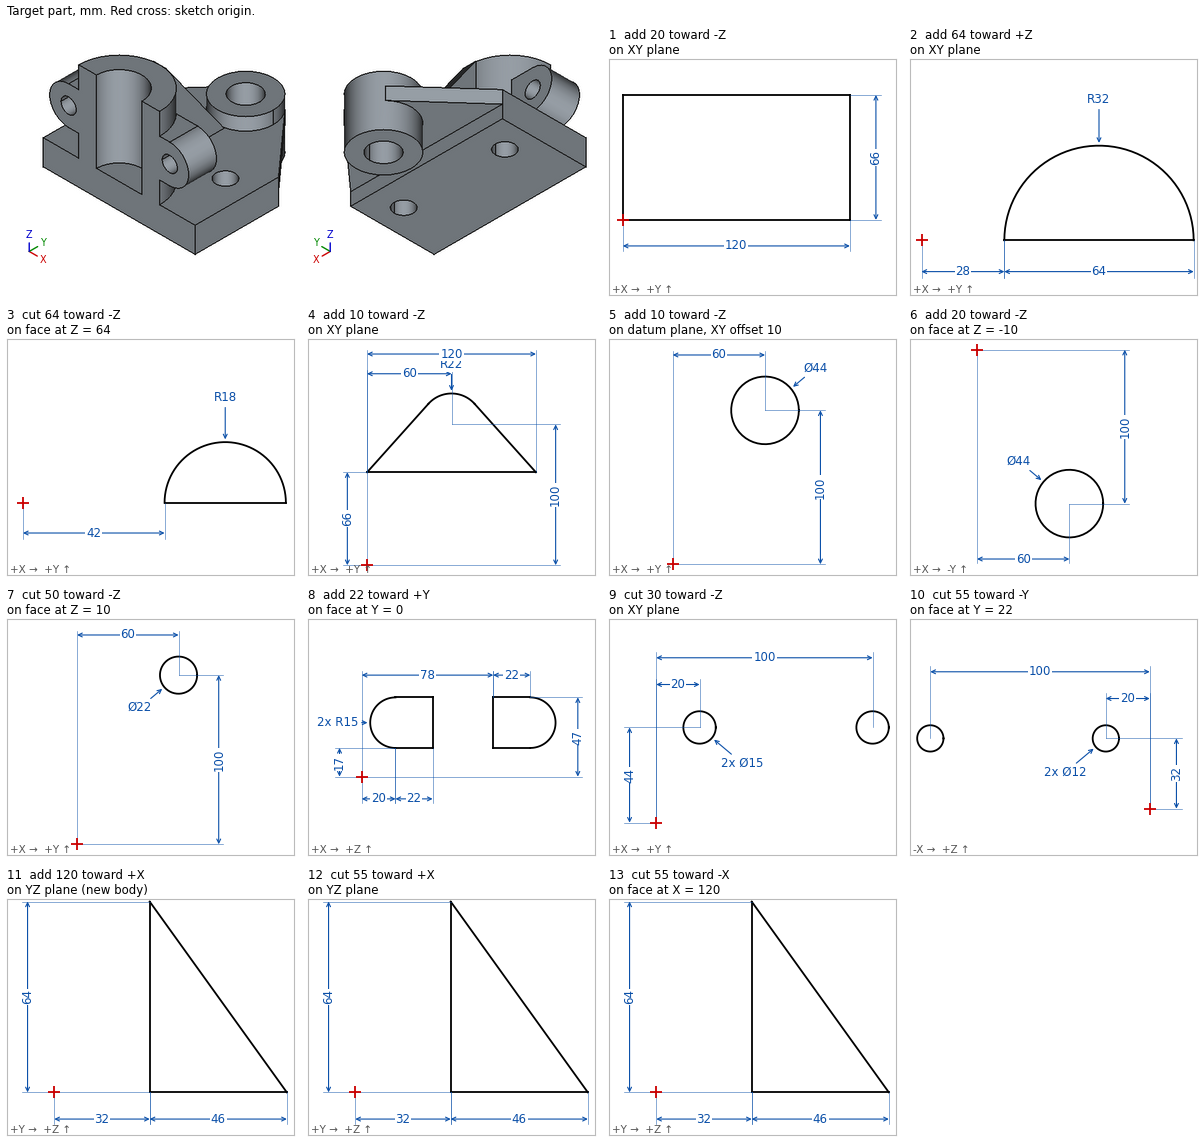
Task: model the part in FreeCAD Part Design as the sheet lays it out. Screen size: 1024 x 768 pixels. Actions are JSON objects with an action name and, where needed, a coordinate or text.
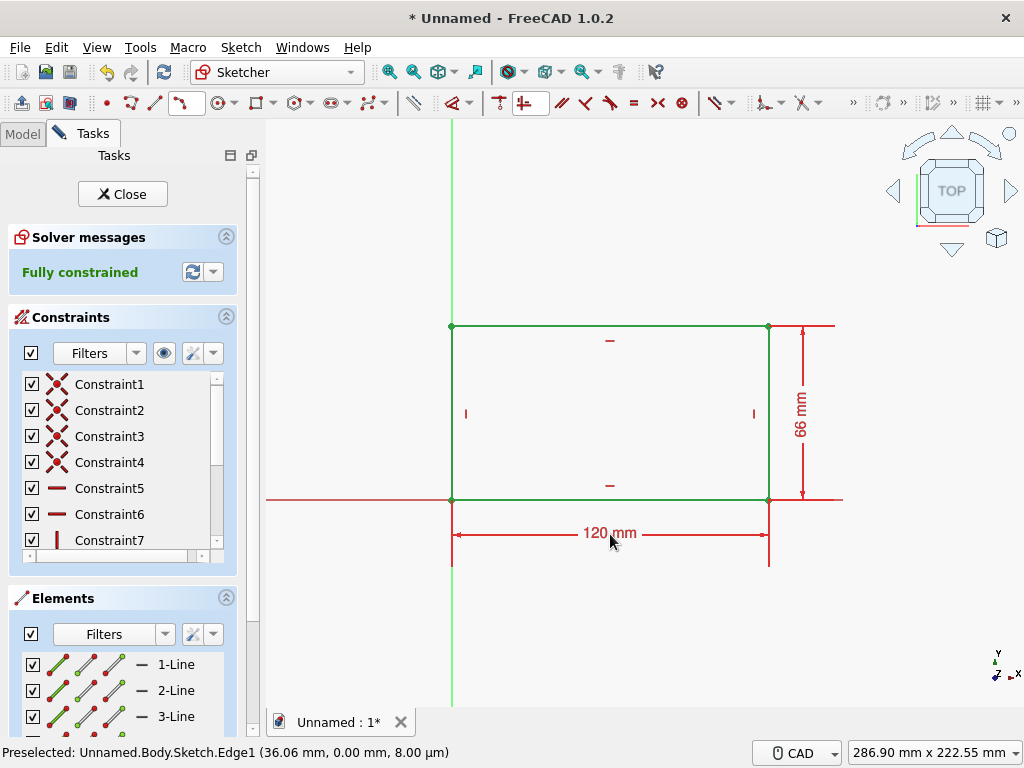
{"action": "left_click", "coordinate": [123, 194]}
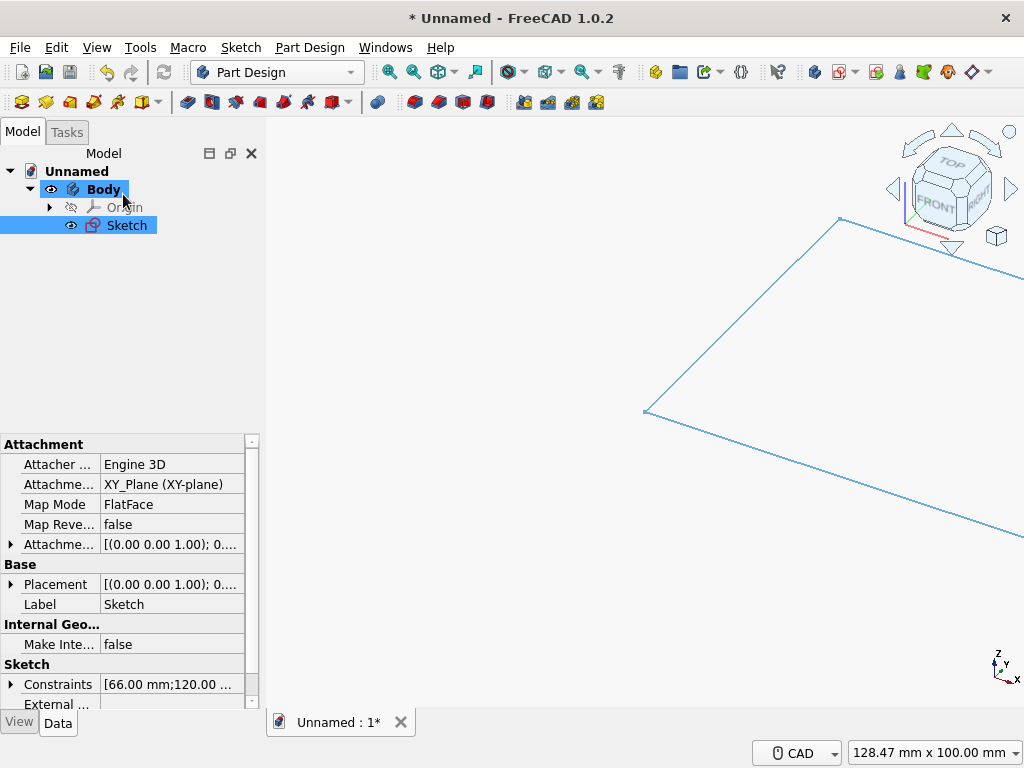
{"action": "left_click", "coordinate": [22, 102]}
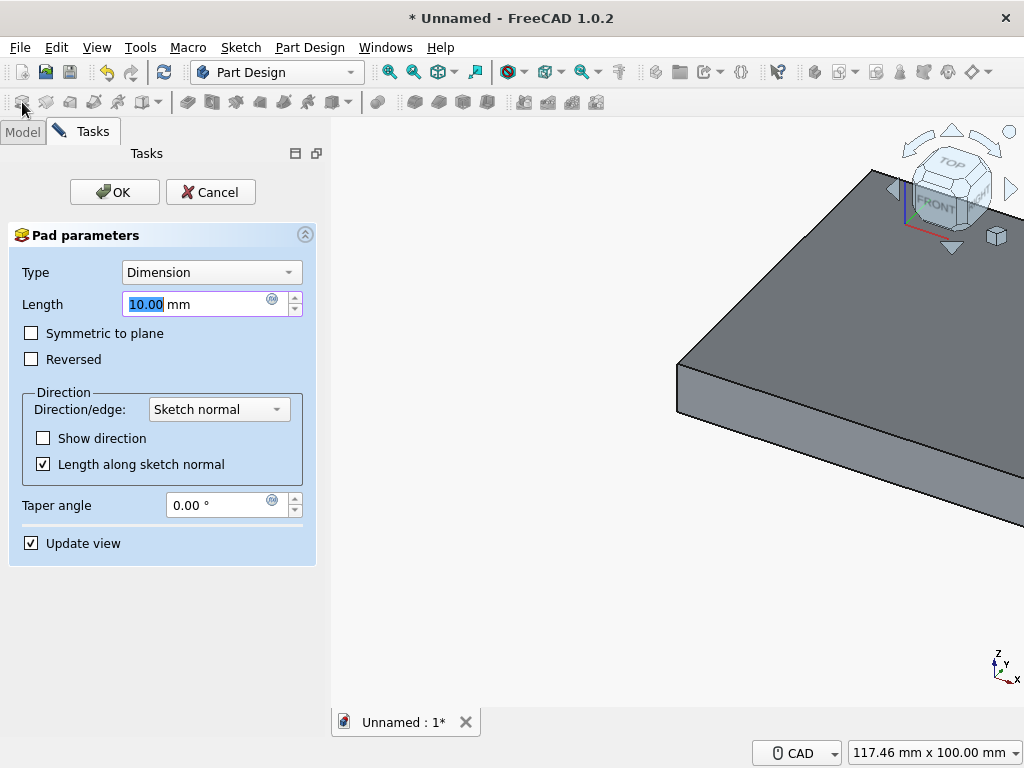
{"action": "type", "text": "20"}
{"action": "key", "text": "Tab"}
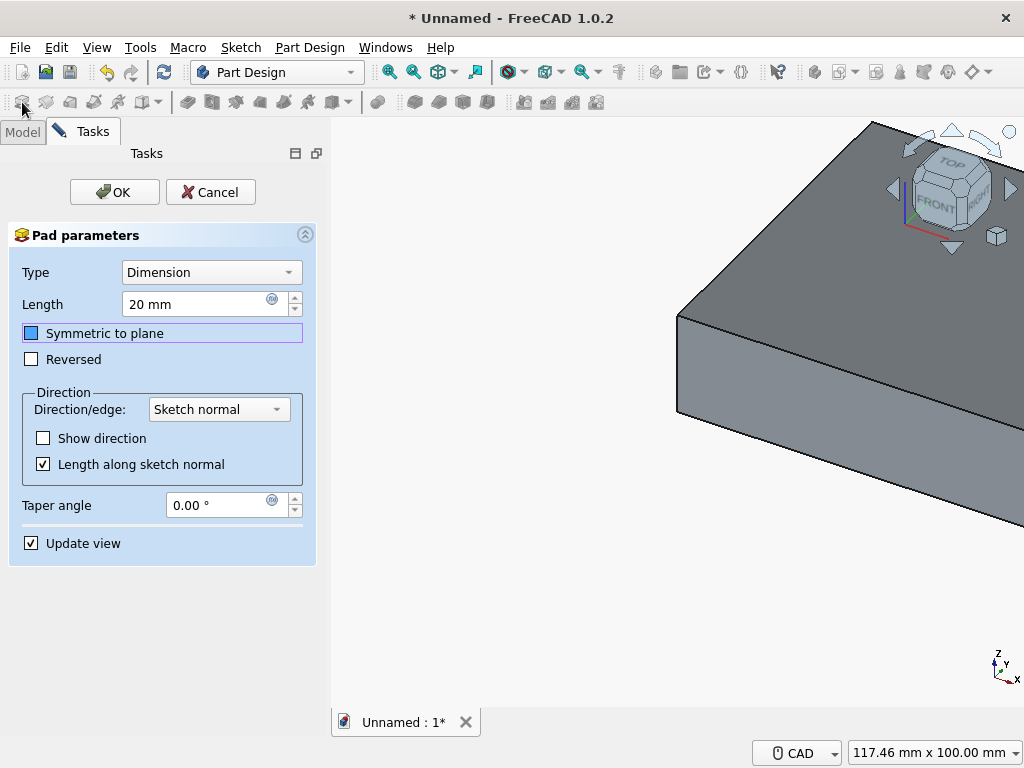
{"action": "left_click", "coordinate": [30, 359]}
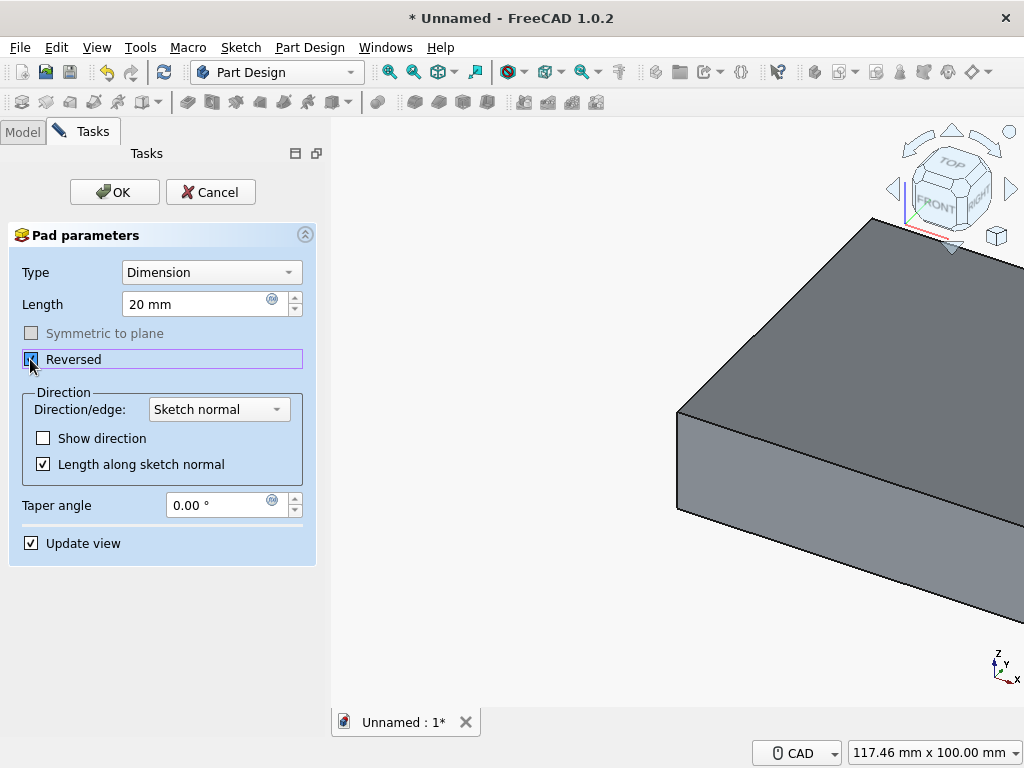
{"action": "left_click", "coordinate": [115, 192]}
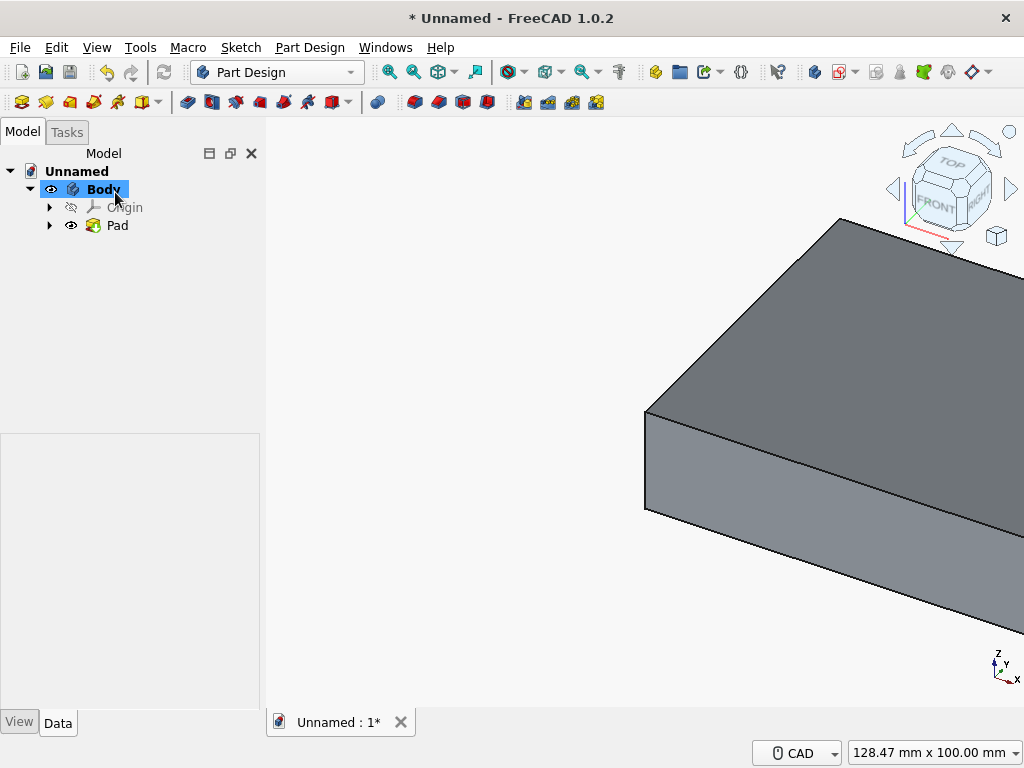
{"action": "left_click", "coordinate": [390, 72]}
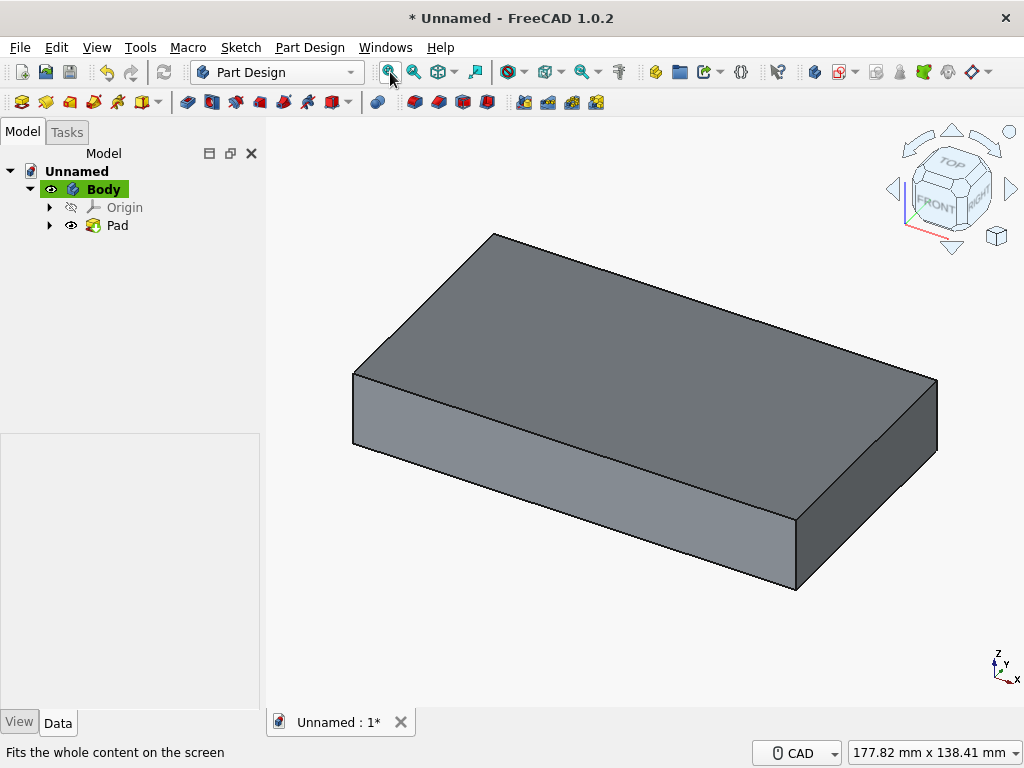
{"action": "left_click", "coordinate": [840, 72]}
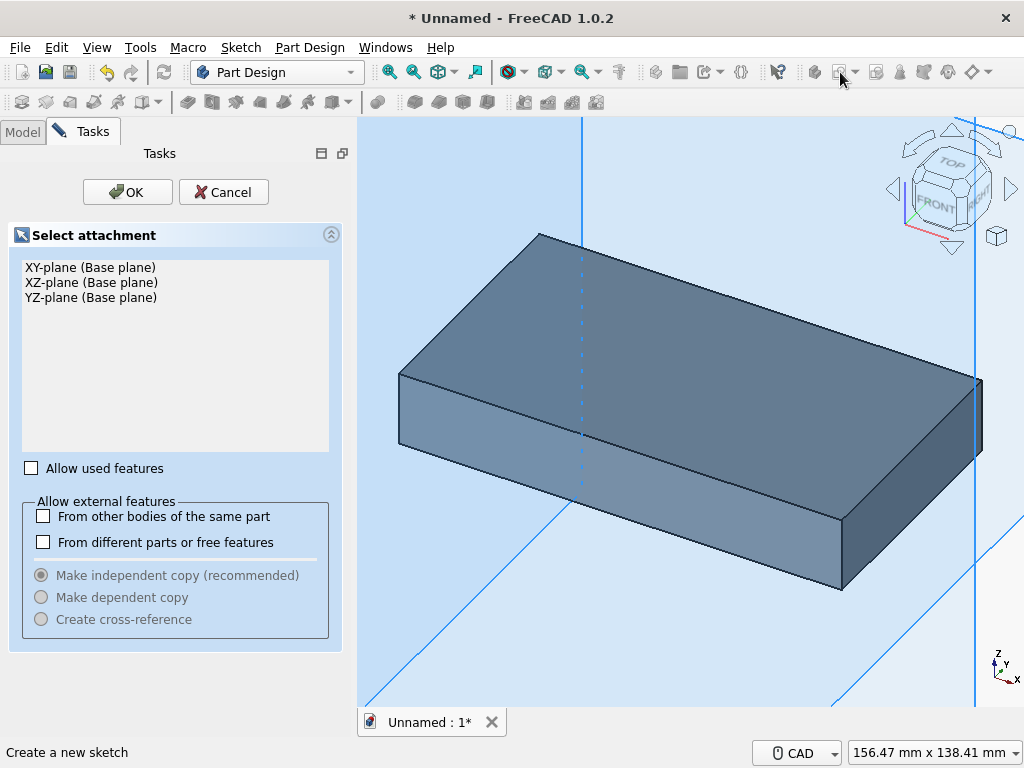
{"action": "left_click", "coordinate": [82, 268]}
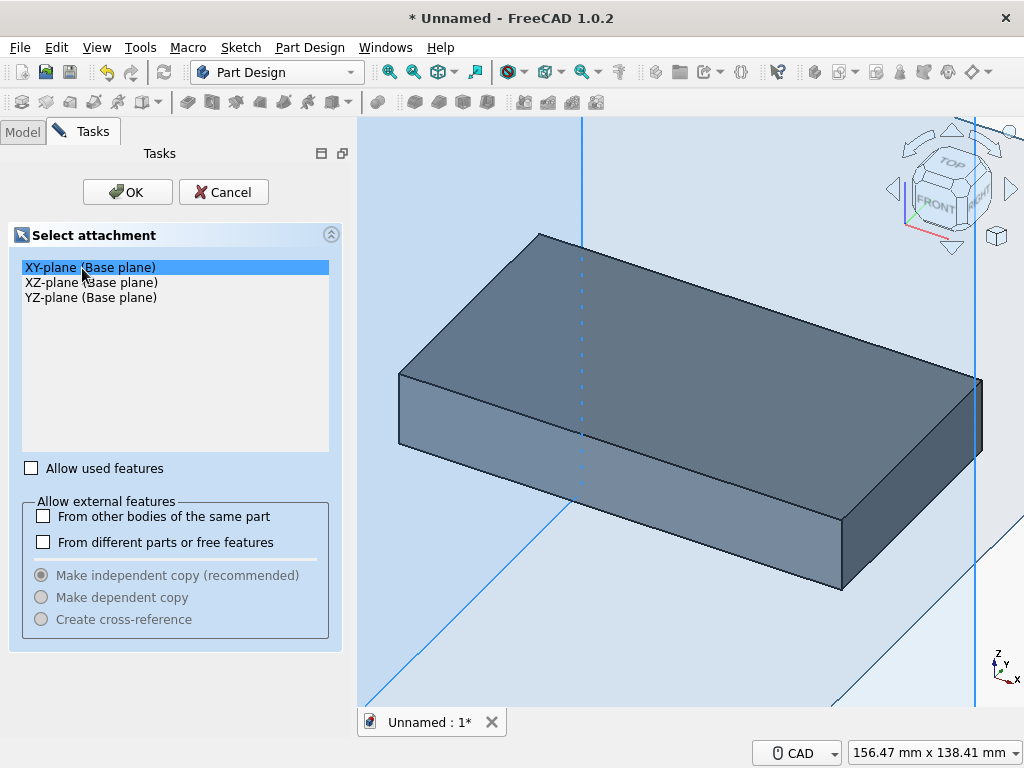
{"action": "left_click", "coordinate": [128, 192]}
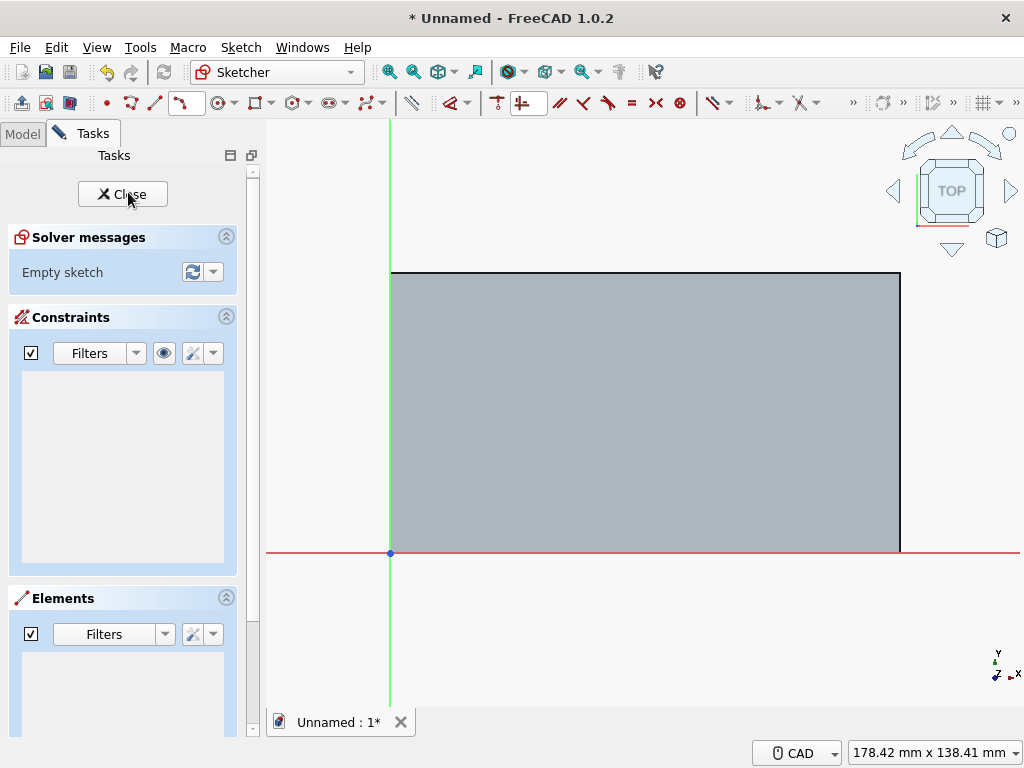
{"action": "left_click", "coordinate": [156, 104]}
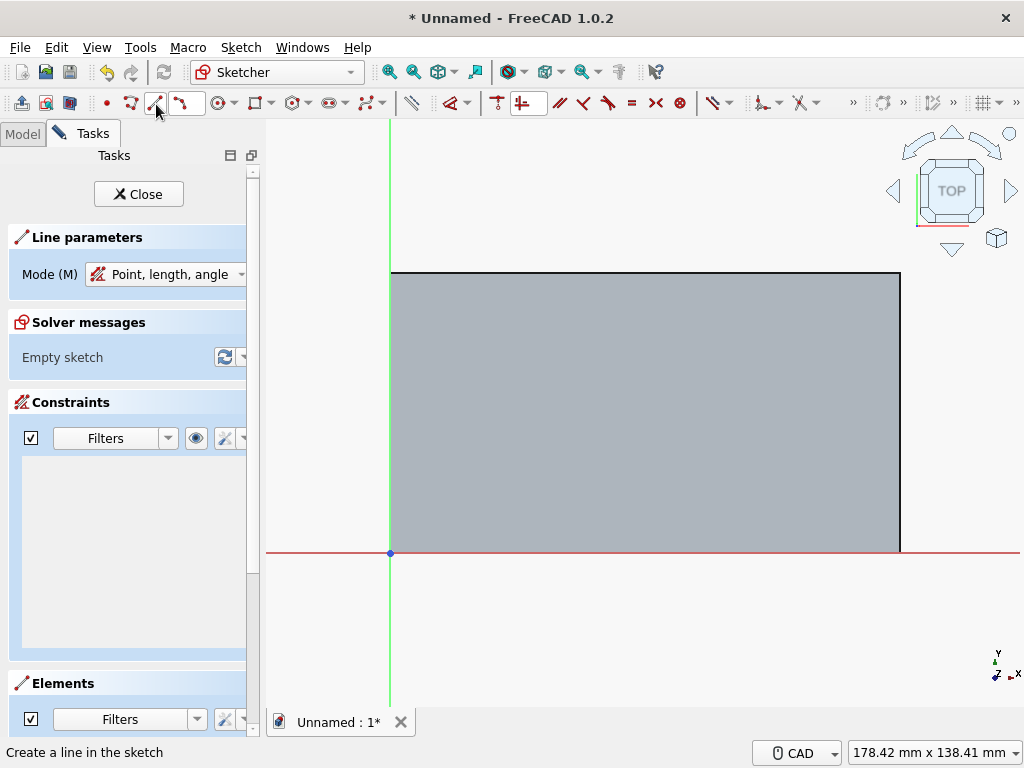
{"action": "left_click", "coordinate": [509, 553]}
{"action": "left_click", "coordinate": [781, 544]}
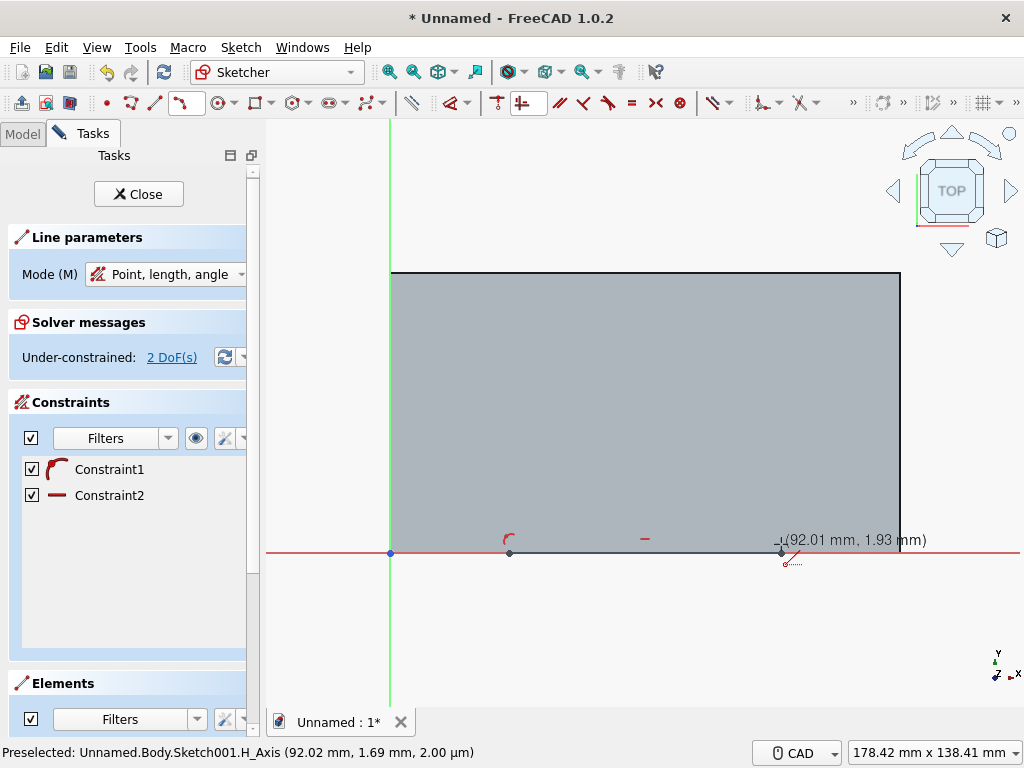
{"action": "left_click", "coordinate": [180, 104]}